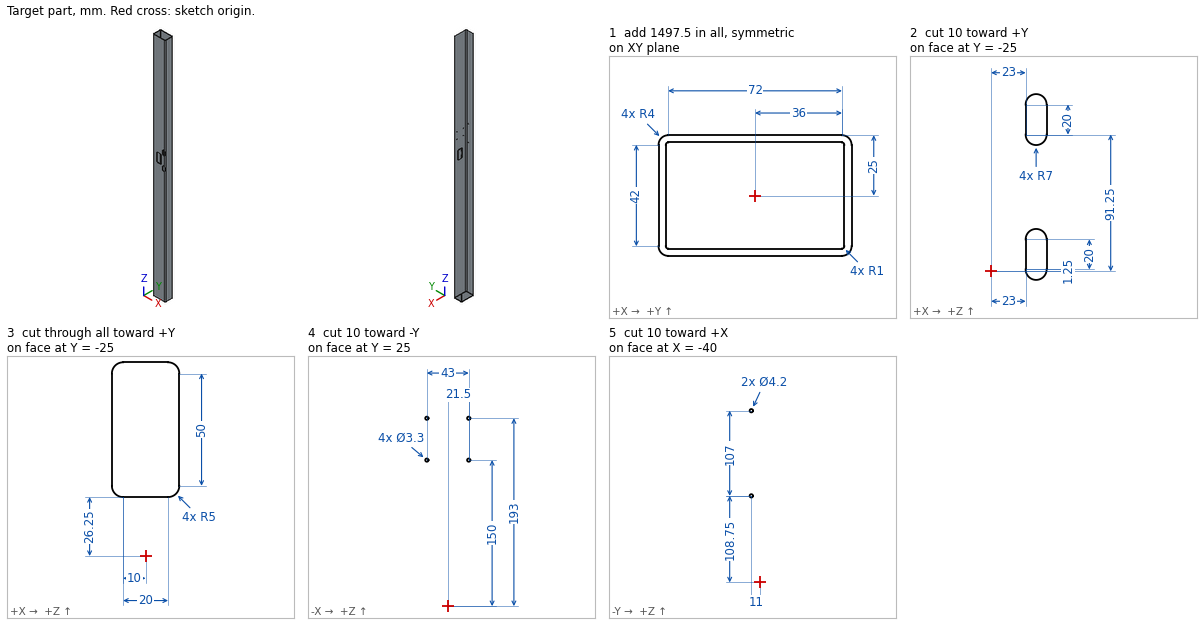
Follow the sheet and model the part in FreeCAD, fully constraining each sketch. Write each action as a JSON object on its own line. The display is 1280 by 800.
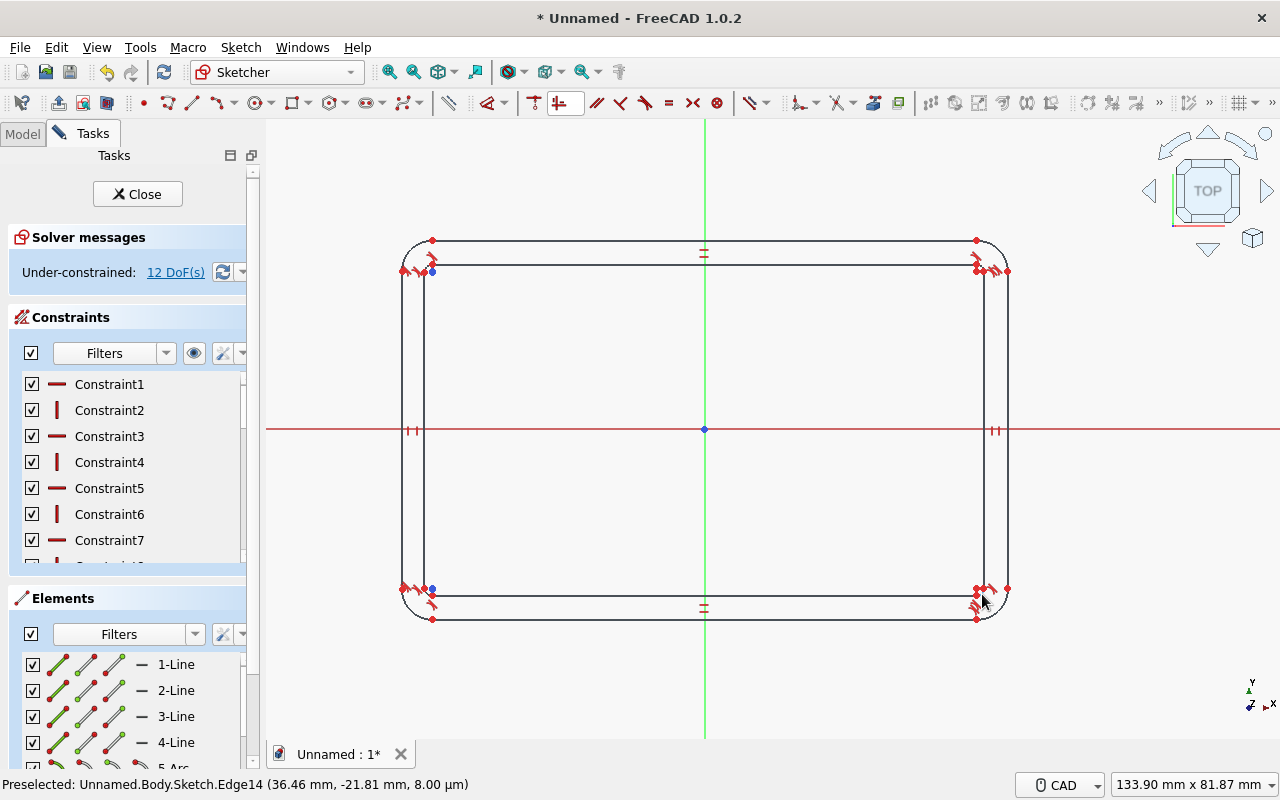
{"action": "left_click", "coordinate": [405, 603]}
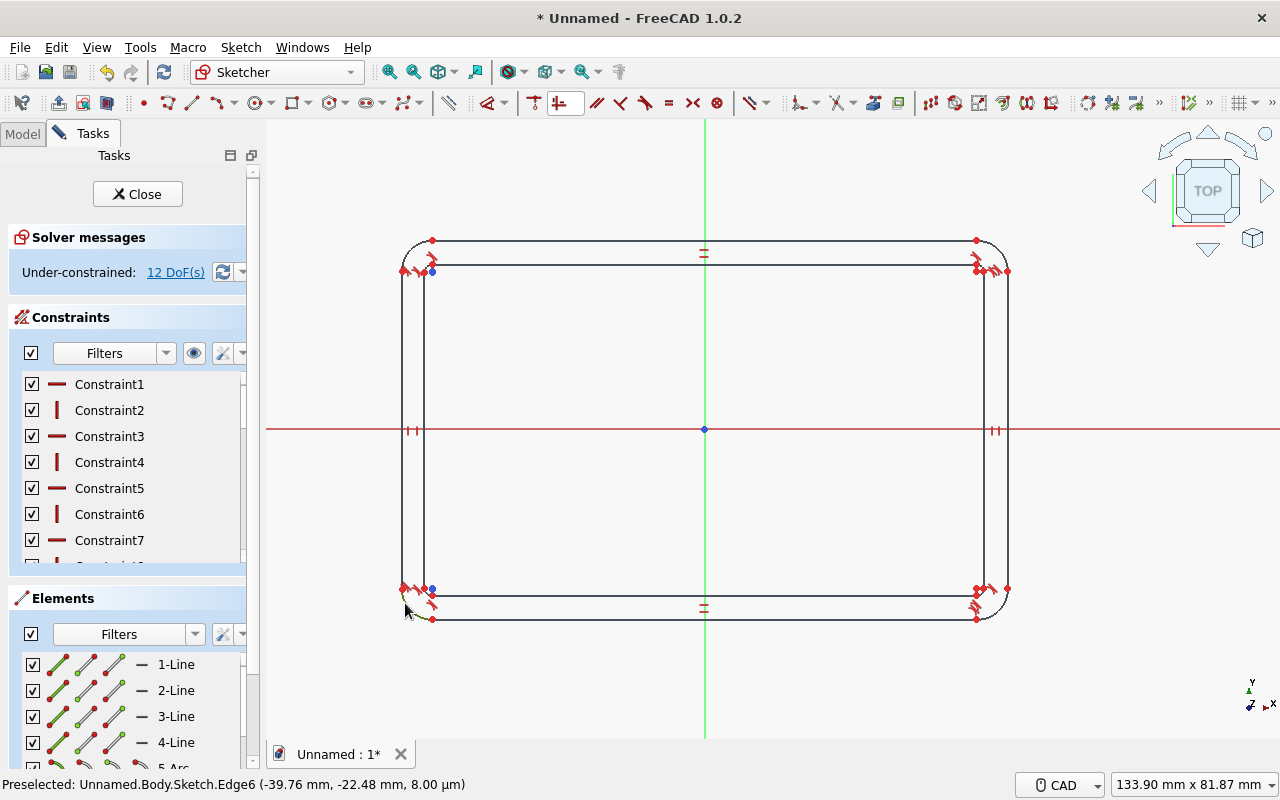
{"action": "scroll", "coordinate": [427, 594], "scroll_direction": "up", "scroll_amount": 5}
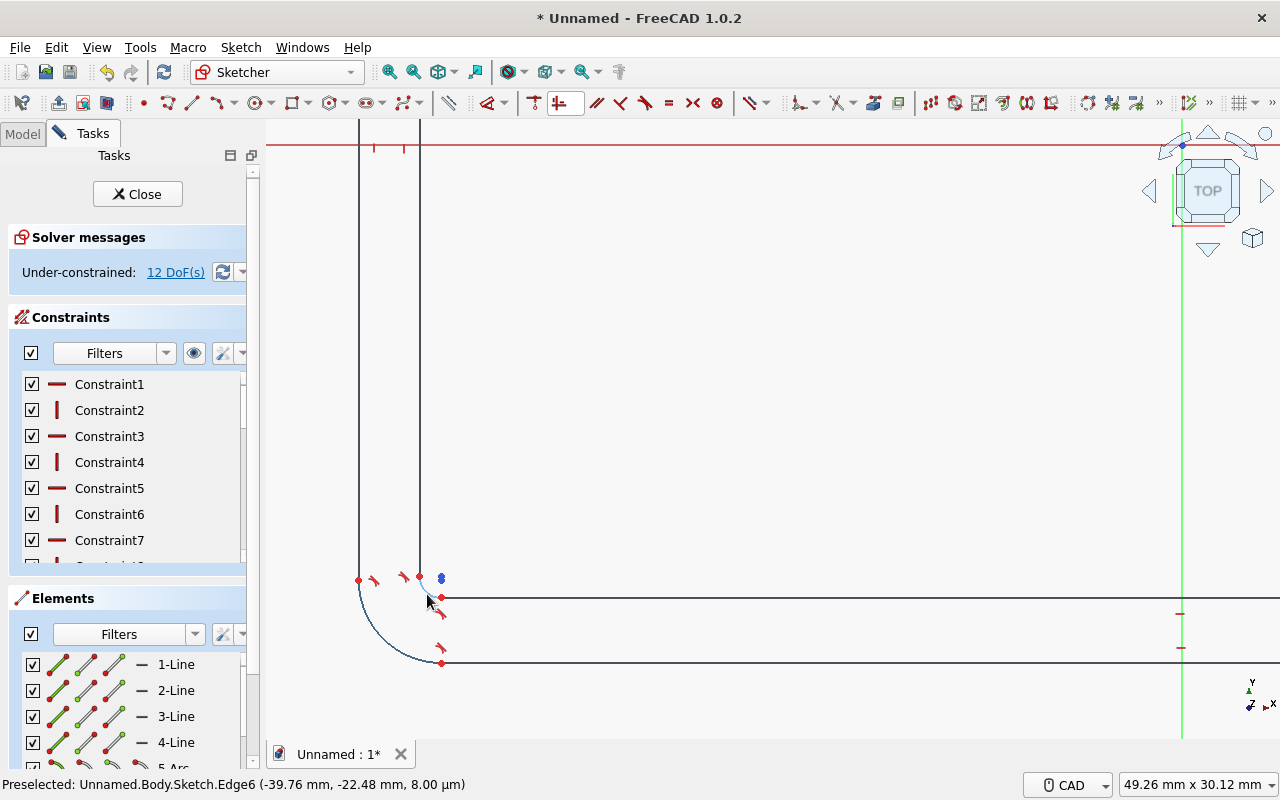
{"action": "left_click", "coordinate": [426, 592]}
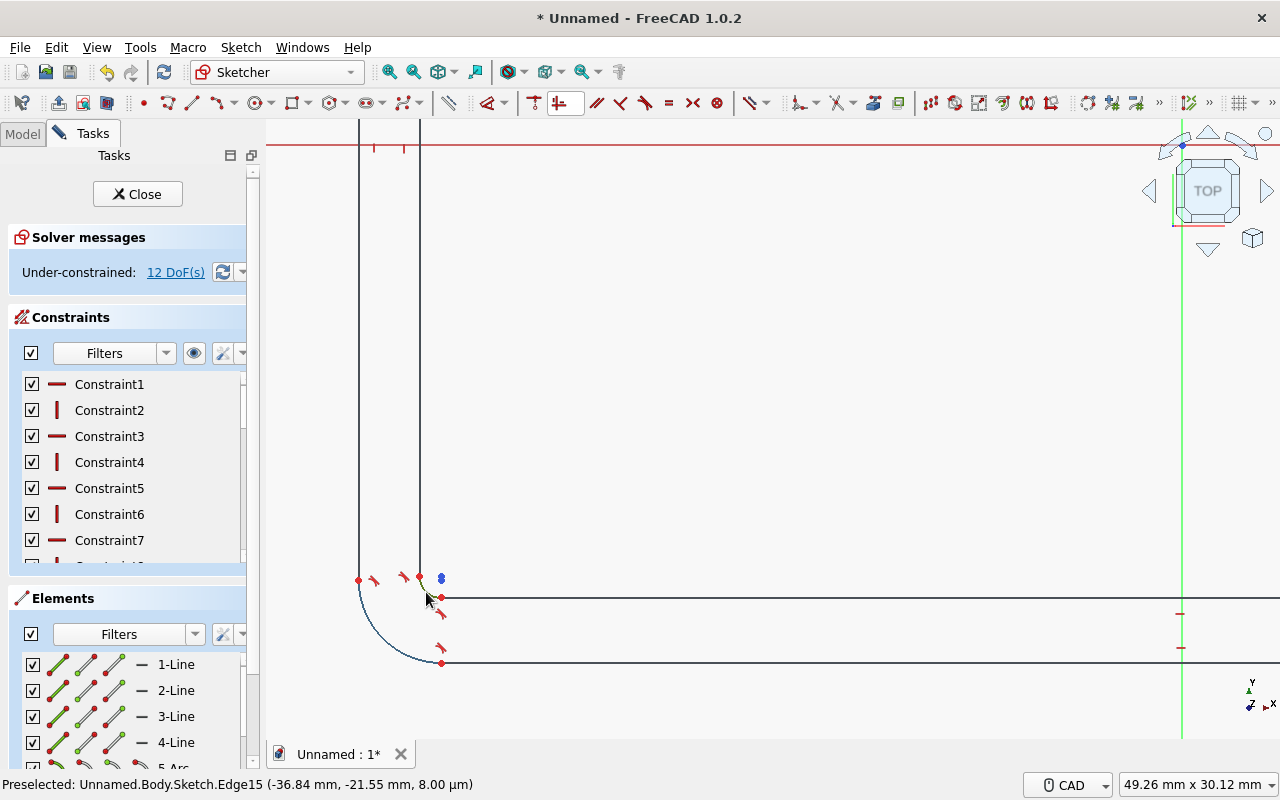
{"action": "key", "text": "c"}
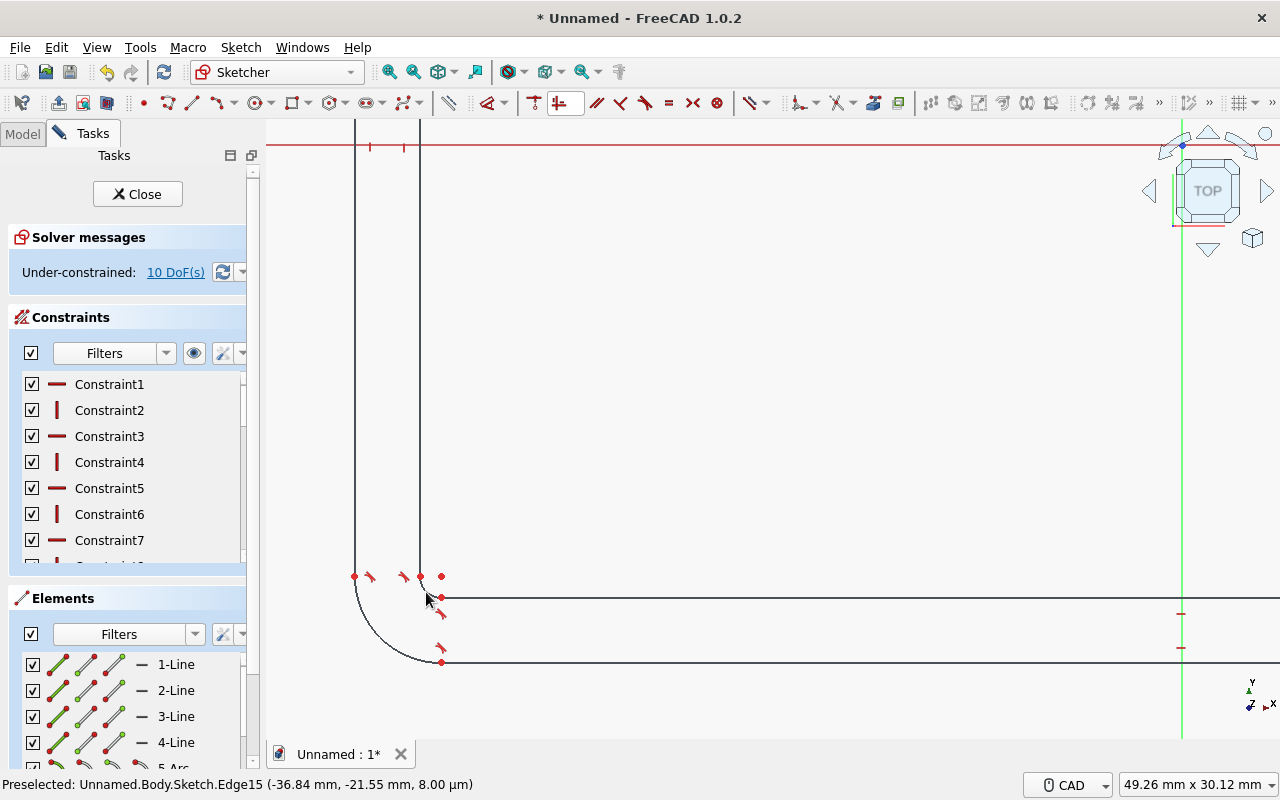
{"action": "scroll", "coordinate": [426, 594], "scroll_direction": "down", "scroll_amount": 5}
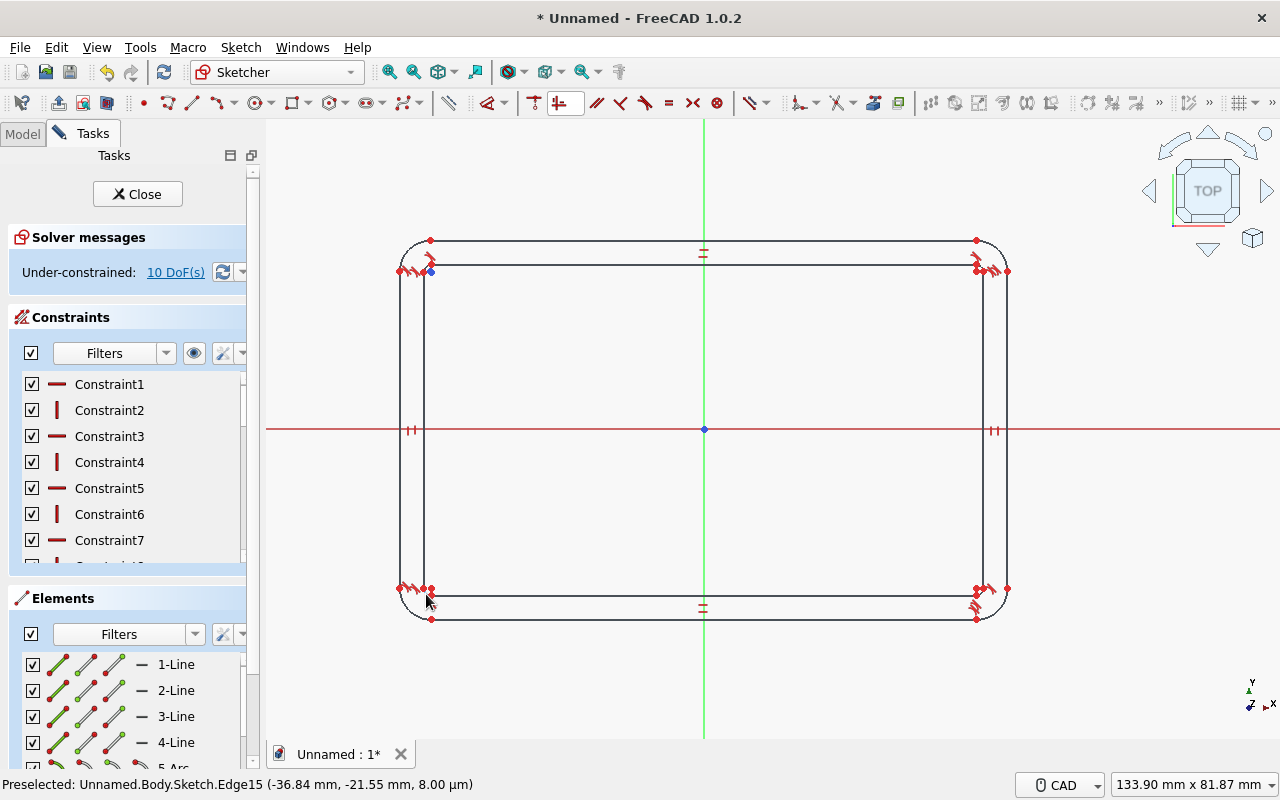
{"action": "left_click", "coordinate": [417, 244]}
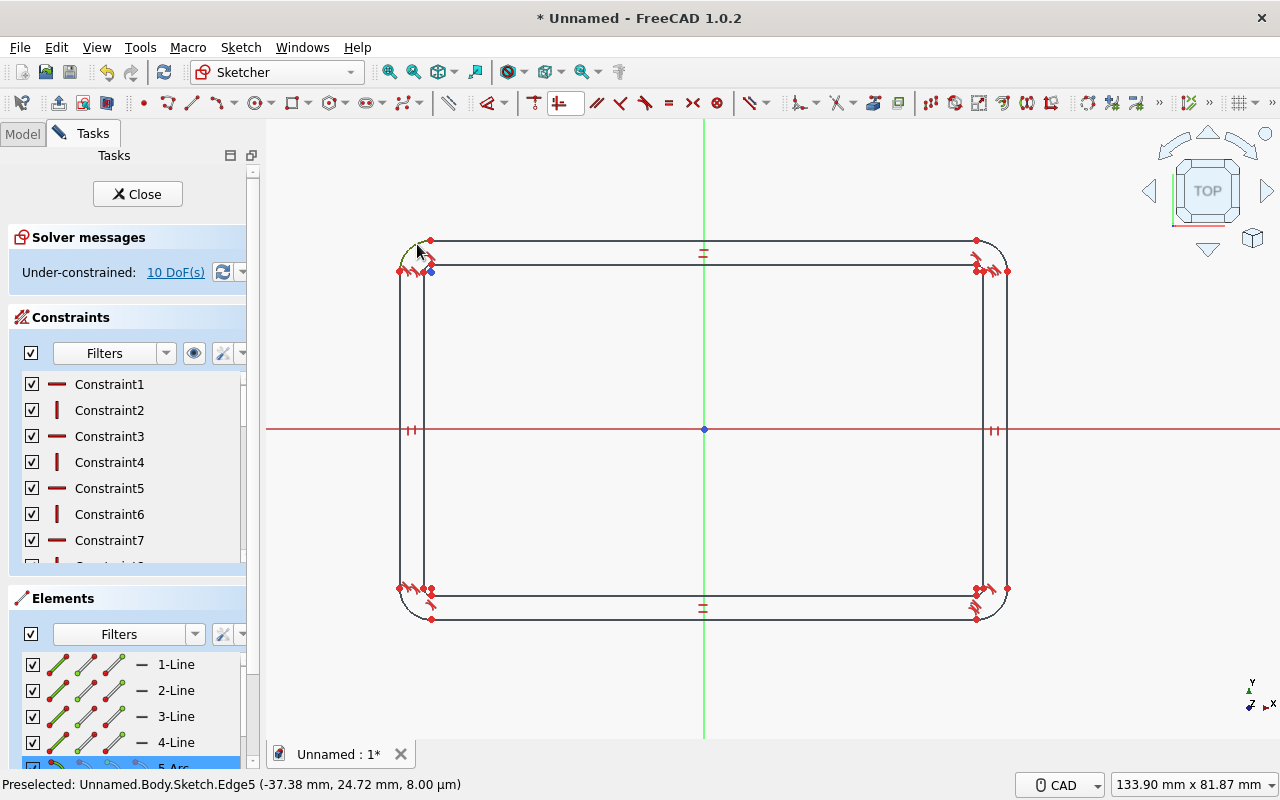
{"action": "left_click", "coordinate": [403, 603]}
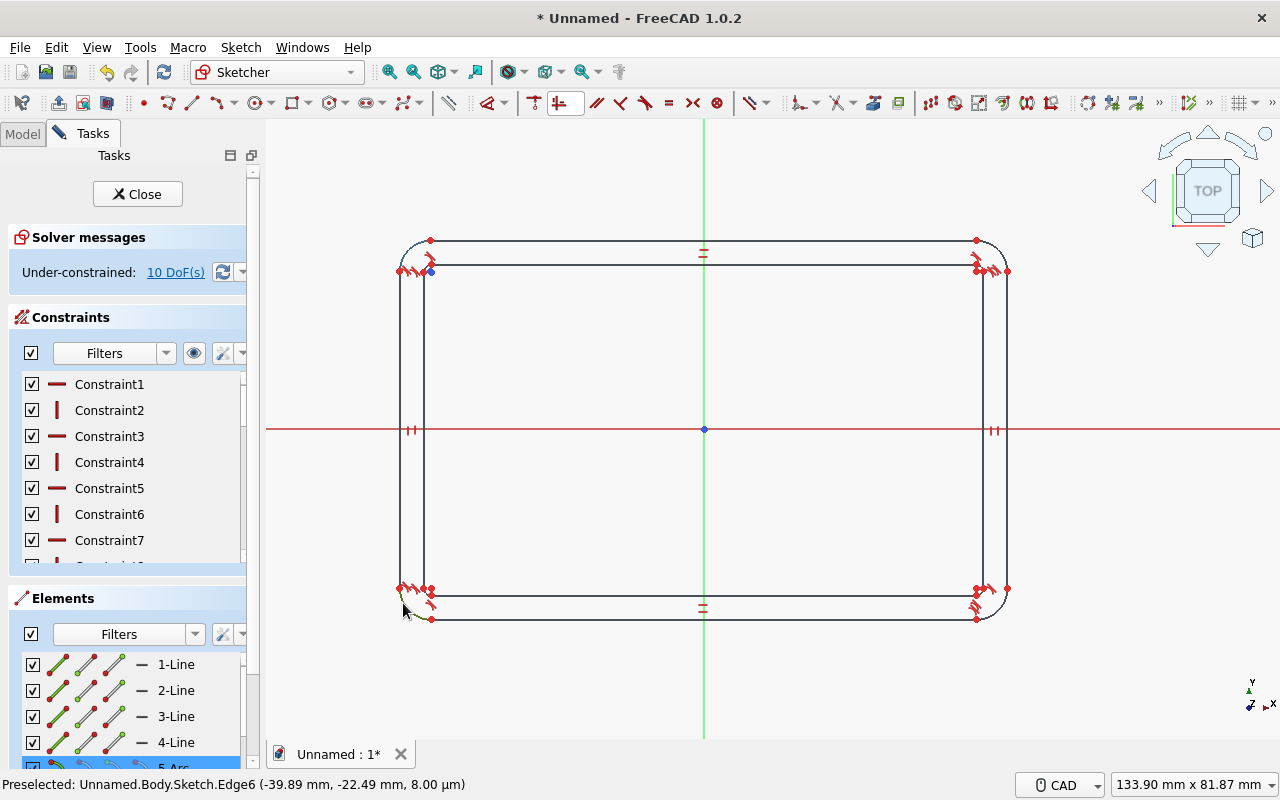
{"action": "left_click", "coordinate": [990, 616]}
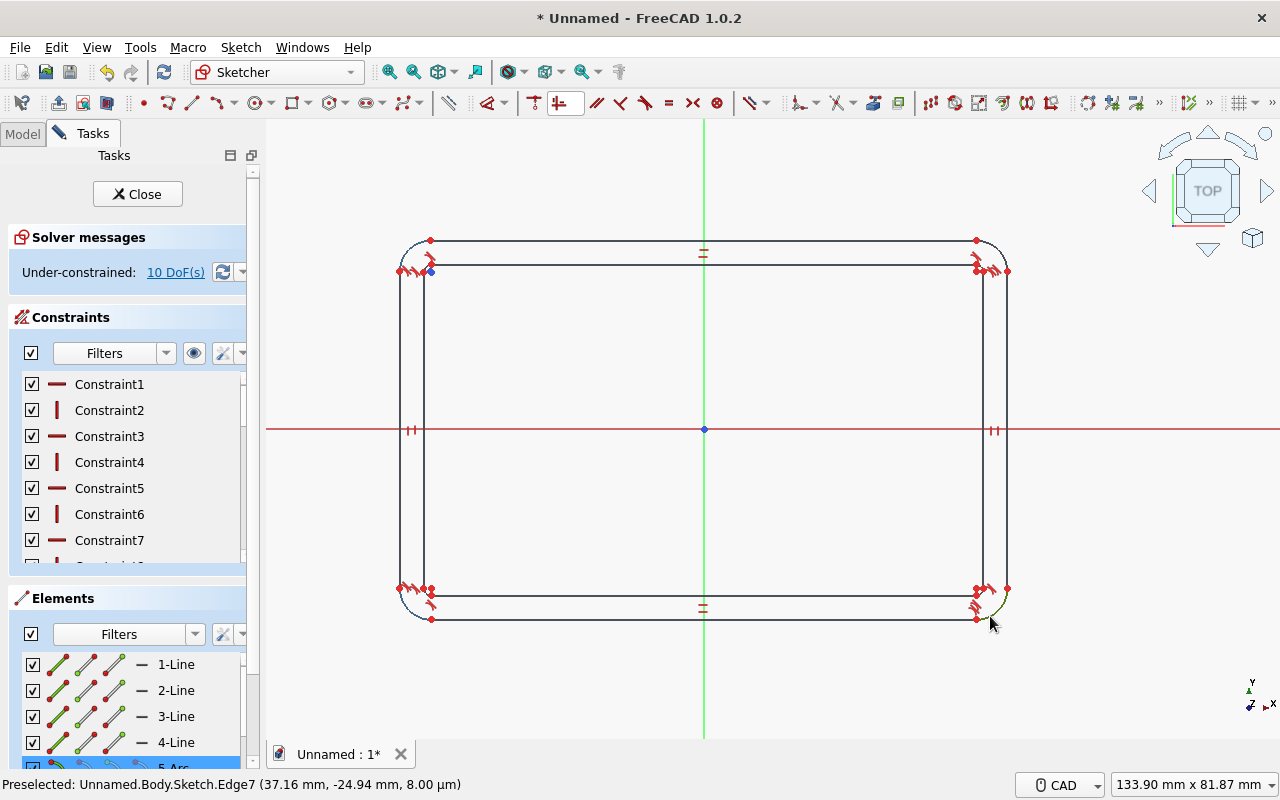
{"action": "left_click", "coordinate": [1004, 258]}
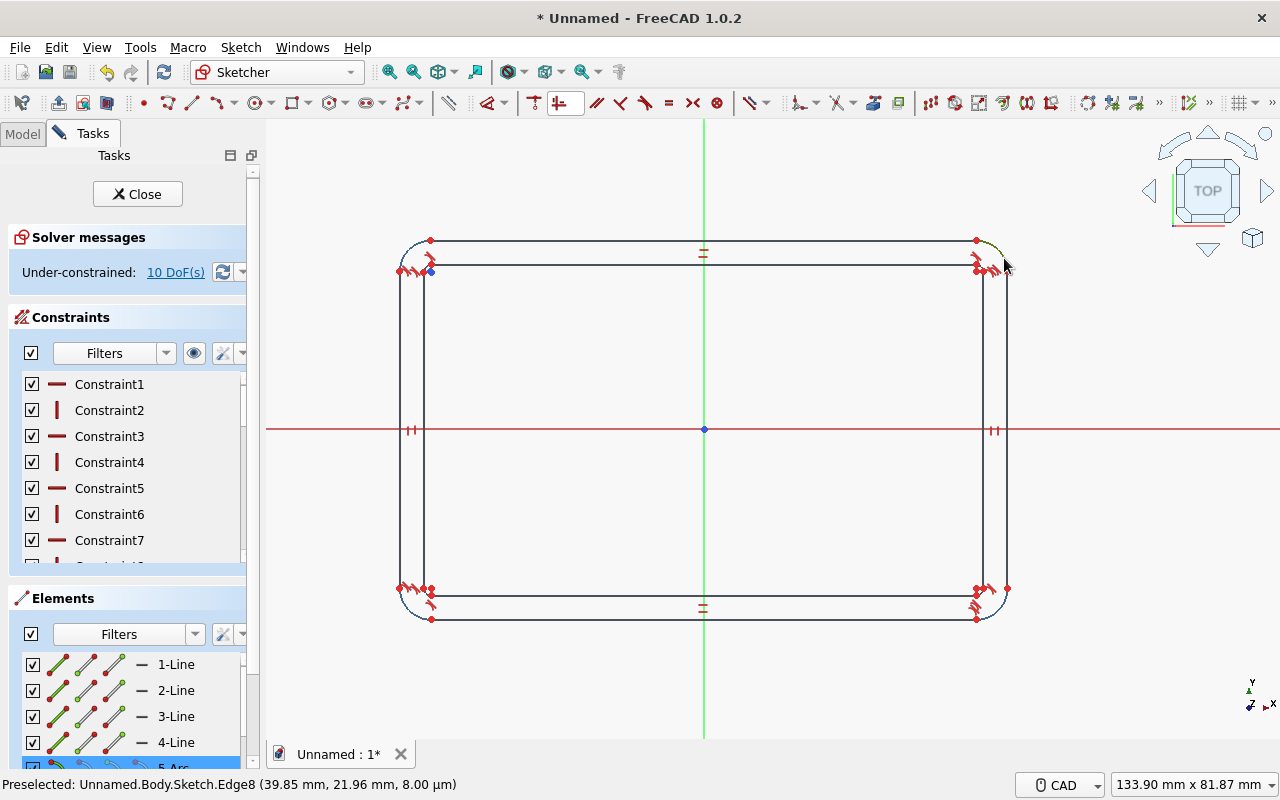
{"action": "key", "text": "e"}